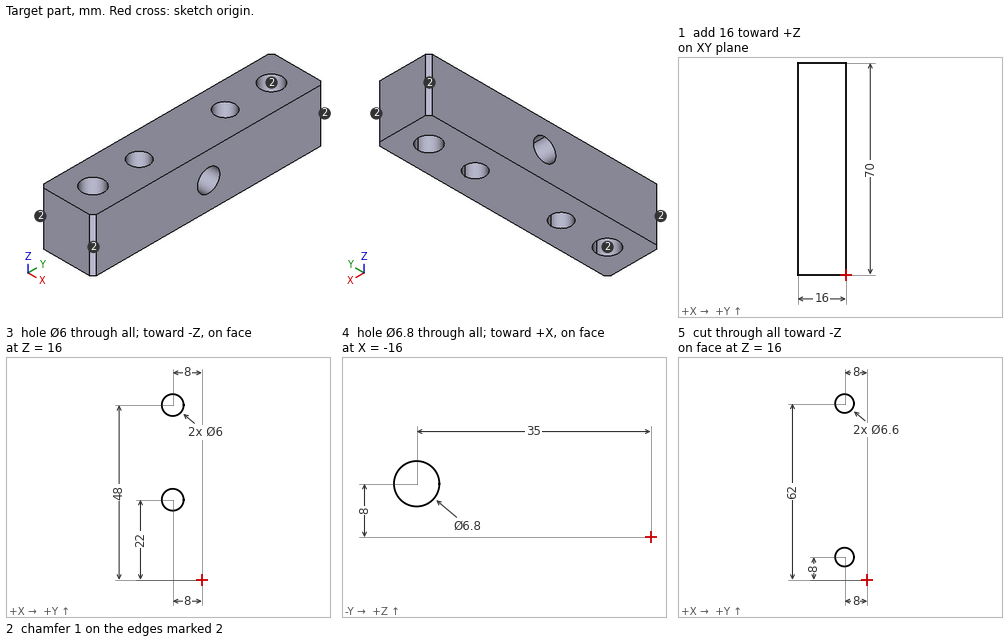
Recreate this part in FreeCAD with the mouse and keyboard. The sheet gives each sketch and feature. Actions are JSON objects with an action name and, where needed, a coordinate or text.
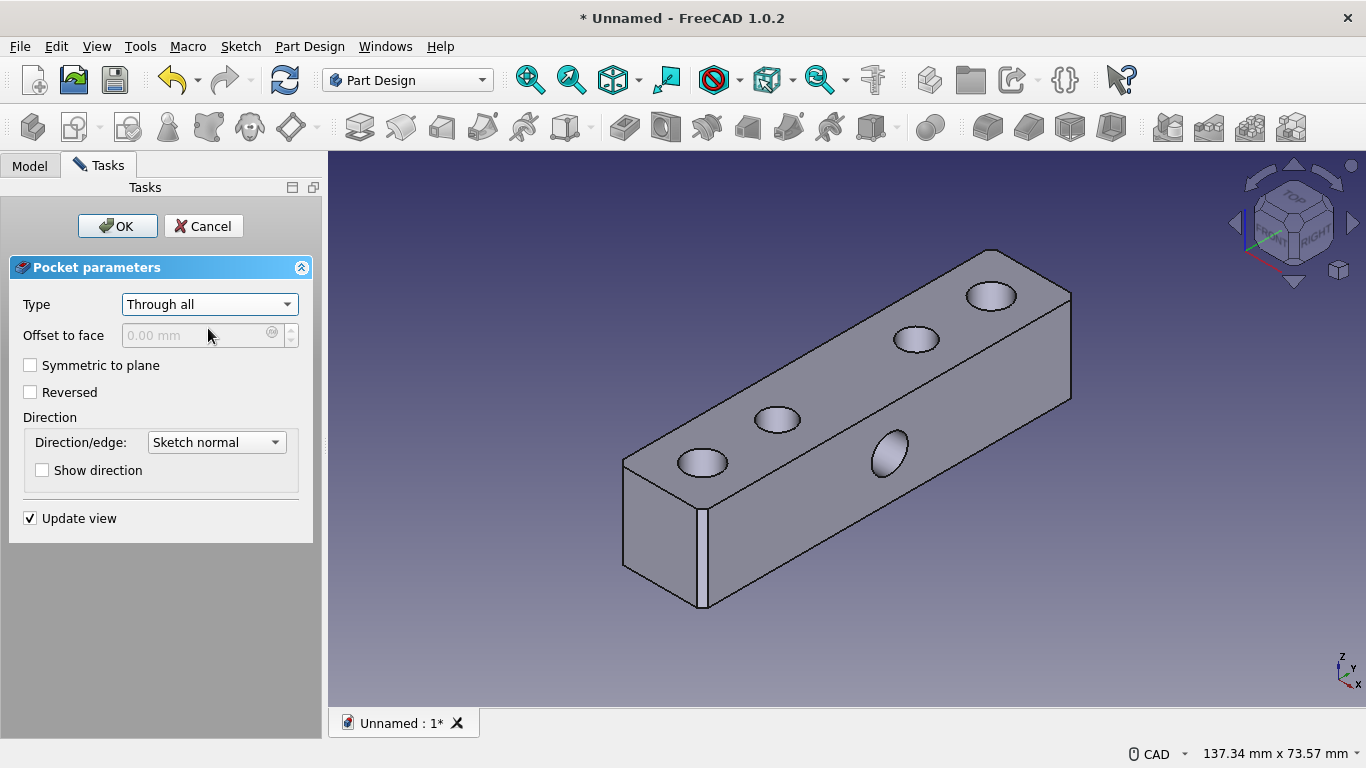
{"action": "left_click", "coordinate": [118, 226]}